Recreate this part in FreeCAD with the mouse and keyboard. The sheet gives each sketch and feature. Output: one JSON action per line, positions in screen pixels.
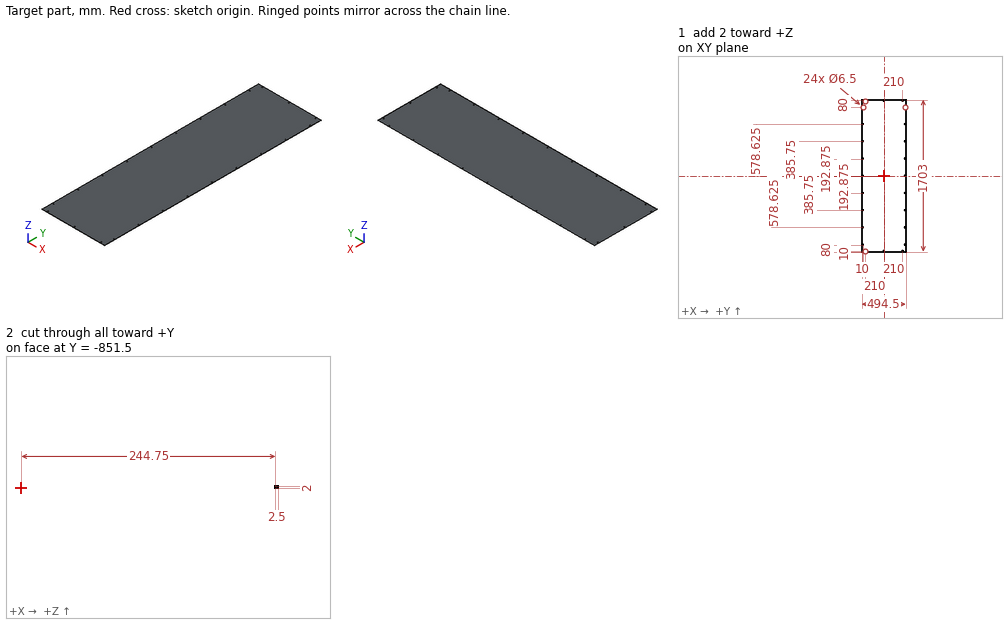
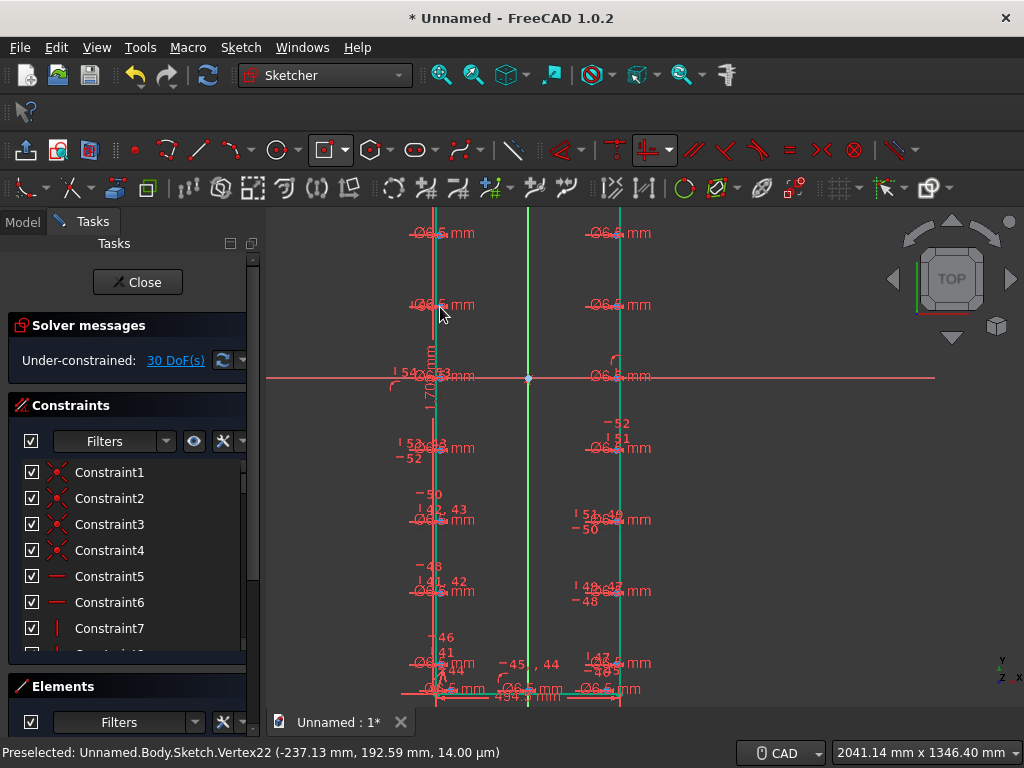
{"action": "left_click", "coordinate": [440, 307]}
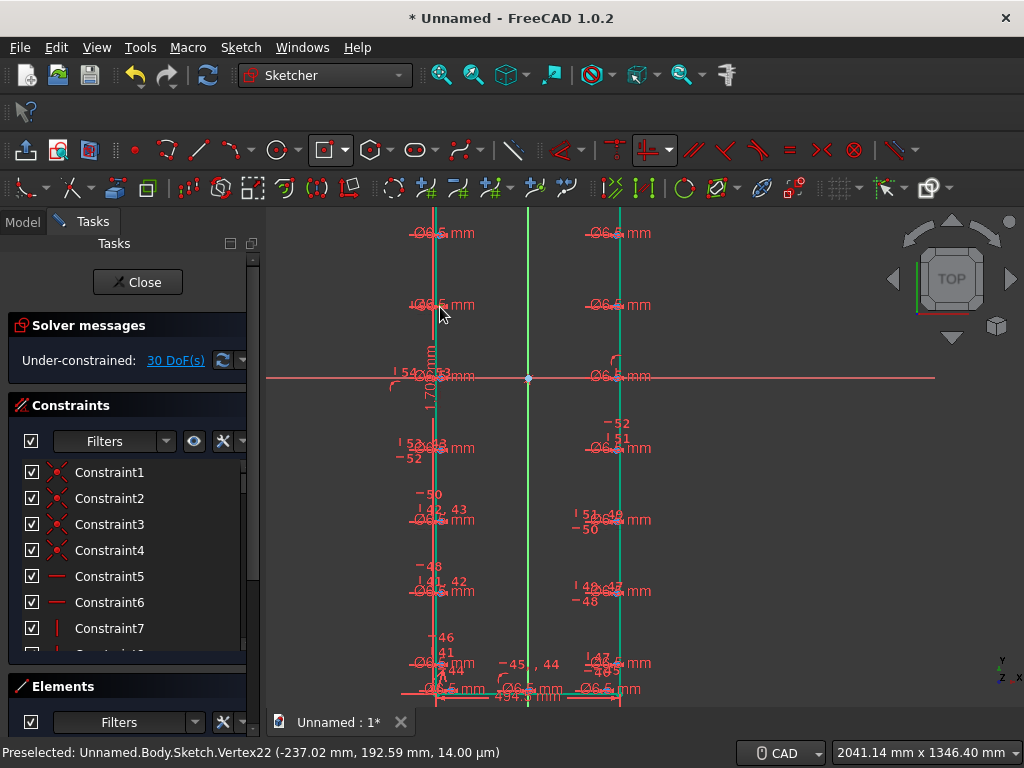
{"action": "left_click", "coordinate": [440, 235]}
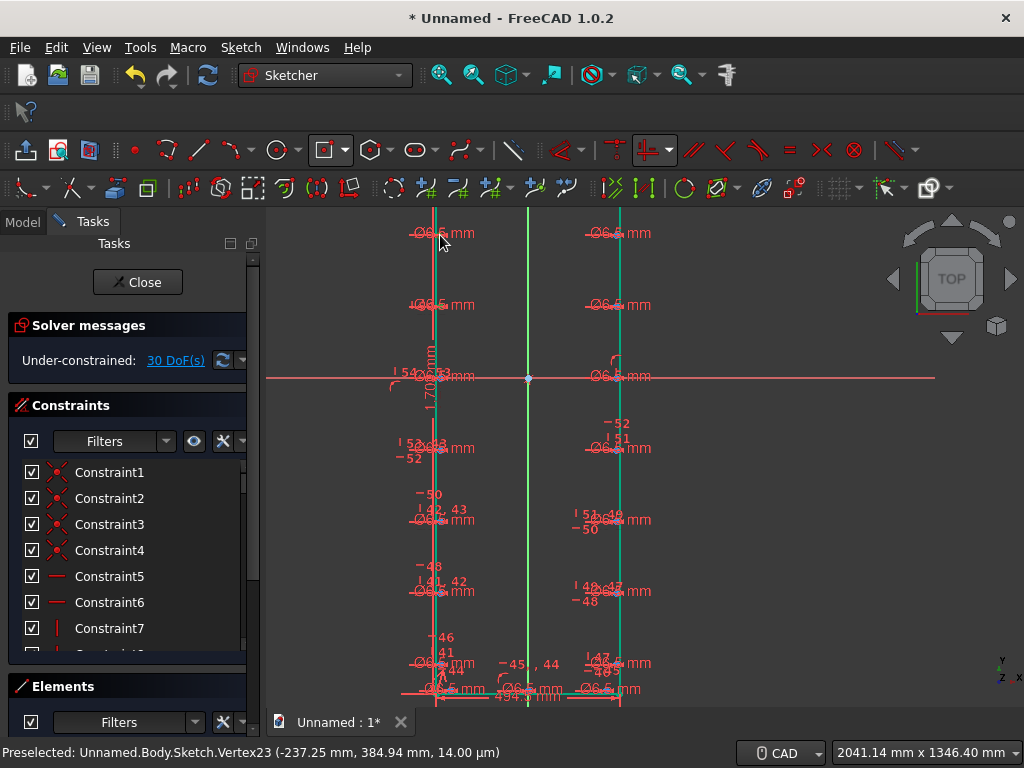
{"action": "key", "text": "v"}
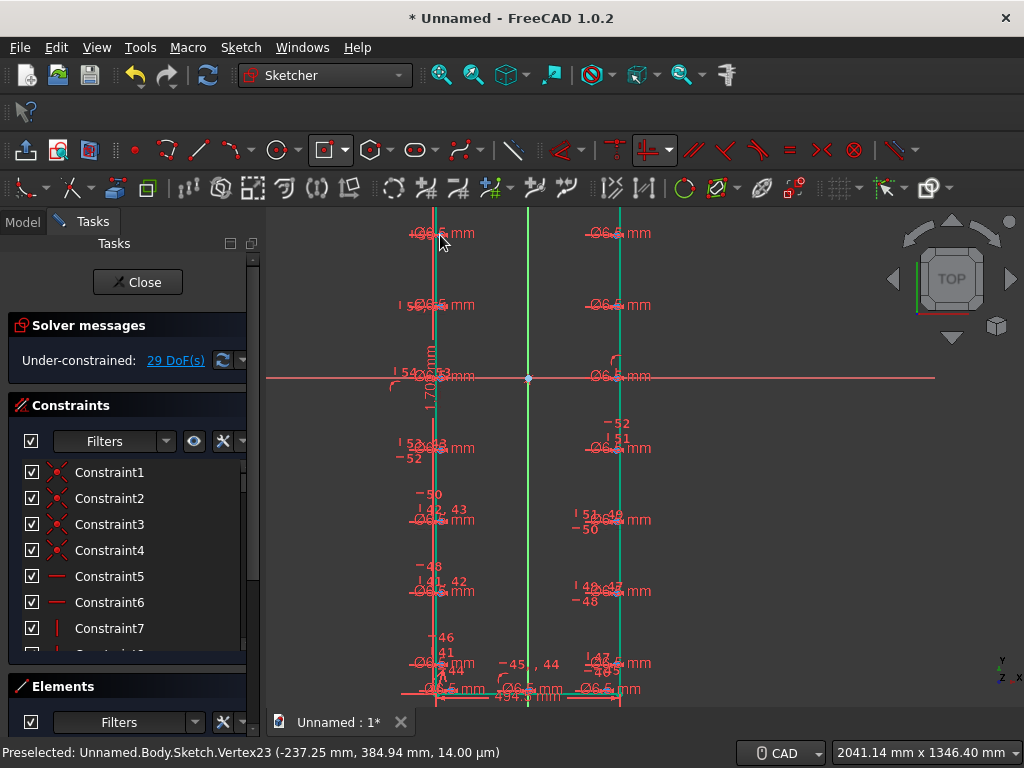
{"action": "left_click", "coordinate": [440, 235]}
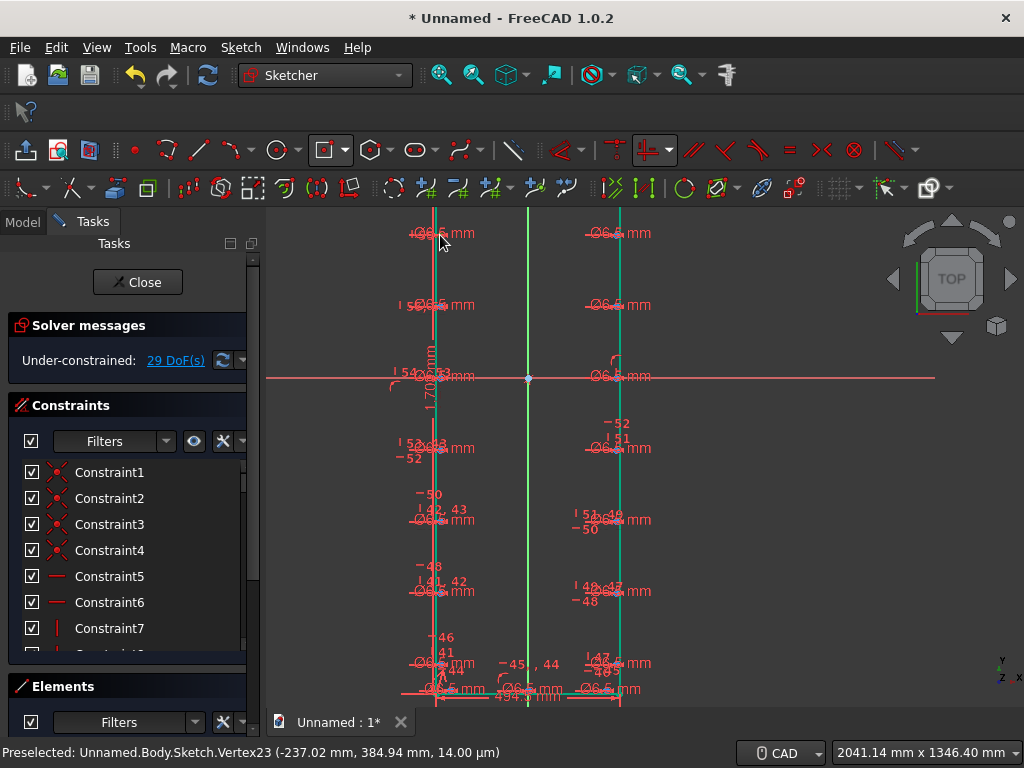
{"action": "scroll", "coordinate": [616, 521], "scroll_direction": "down", "scroll_amount": 4}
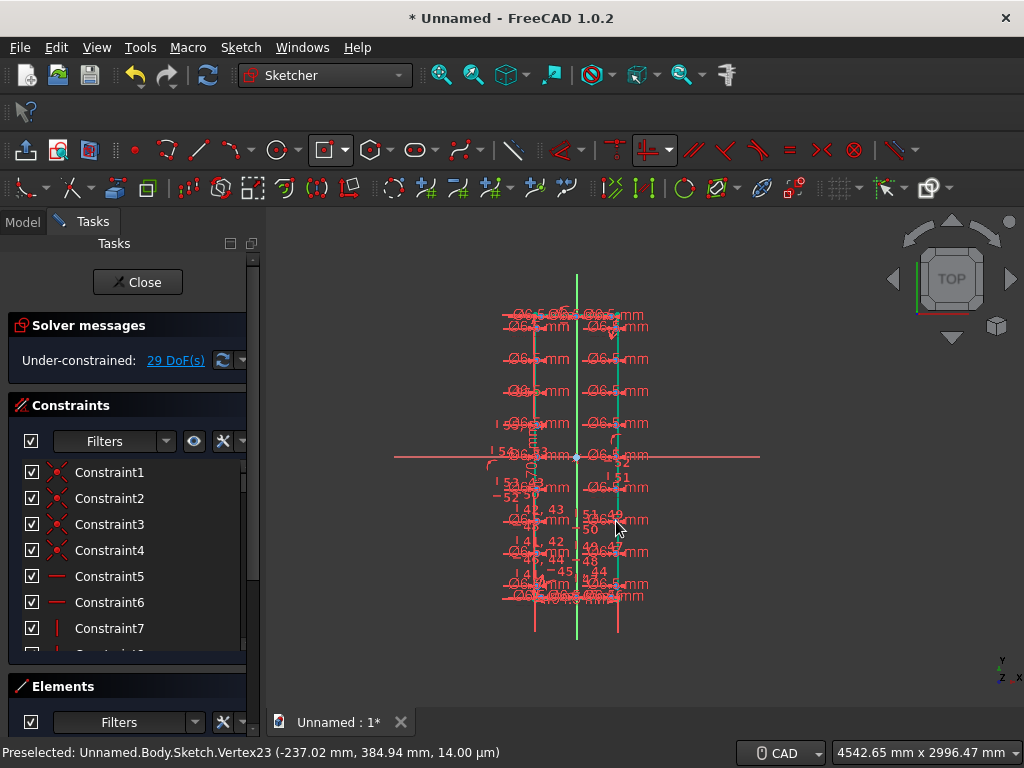
{"action": "left_click", "coordinate": [537, 361]}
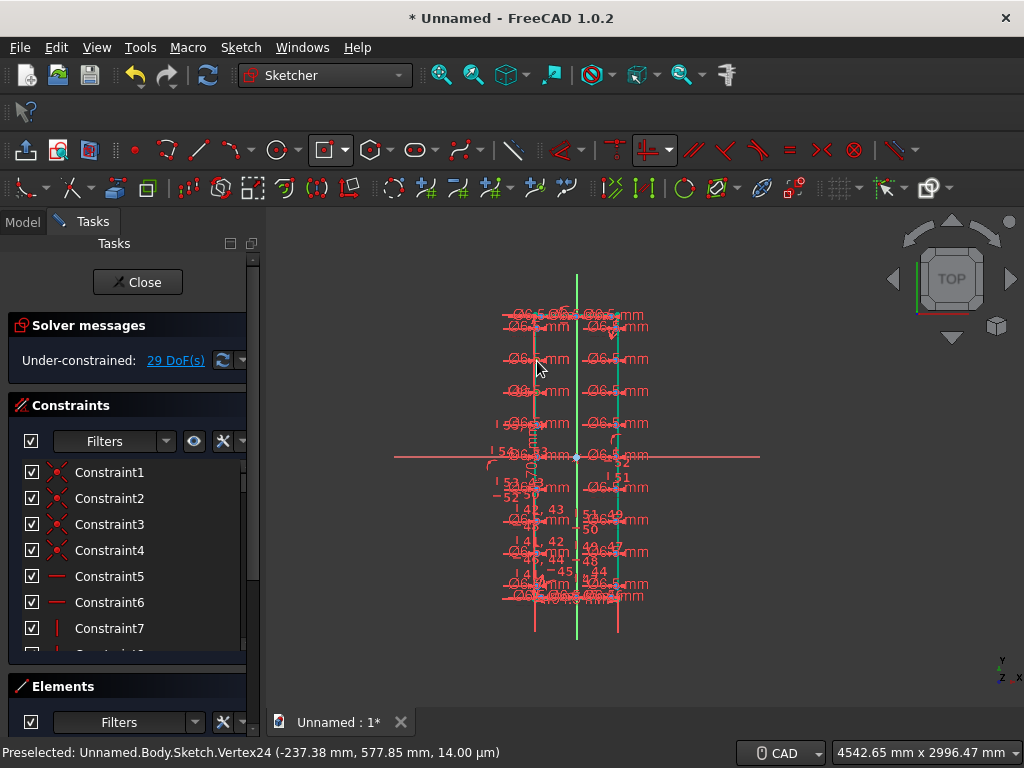
{"action": "key", "text": "v"}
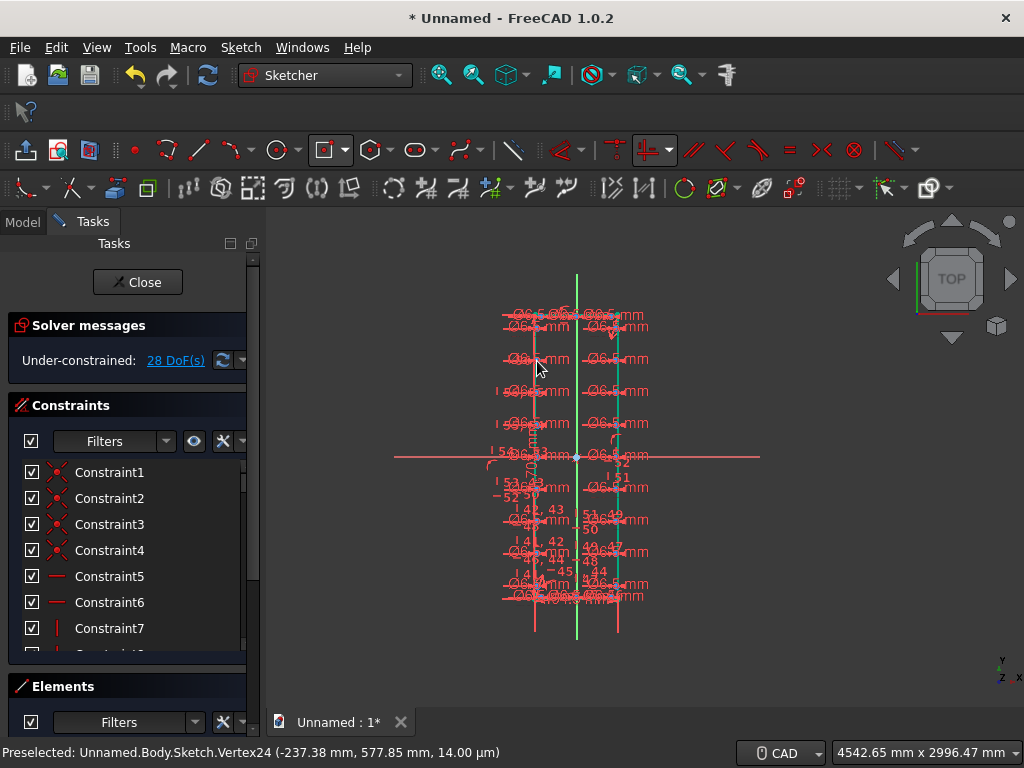
{"action": "left_click", "coordinate": [537, 361]}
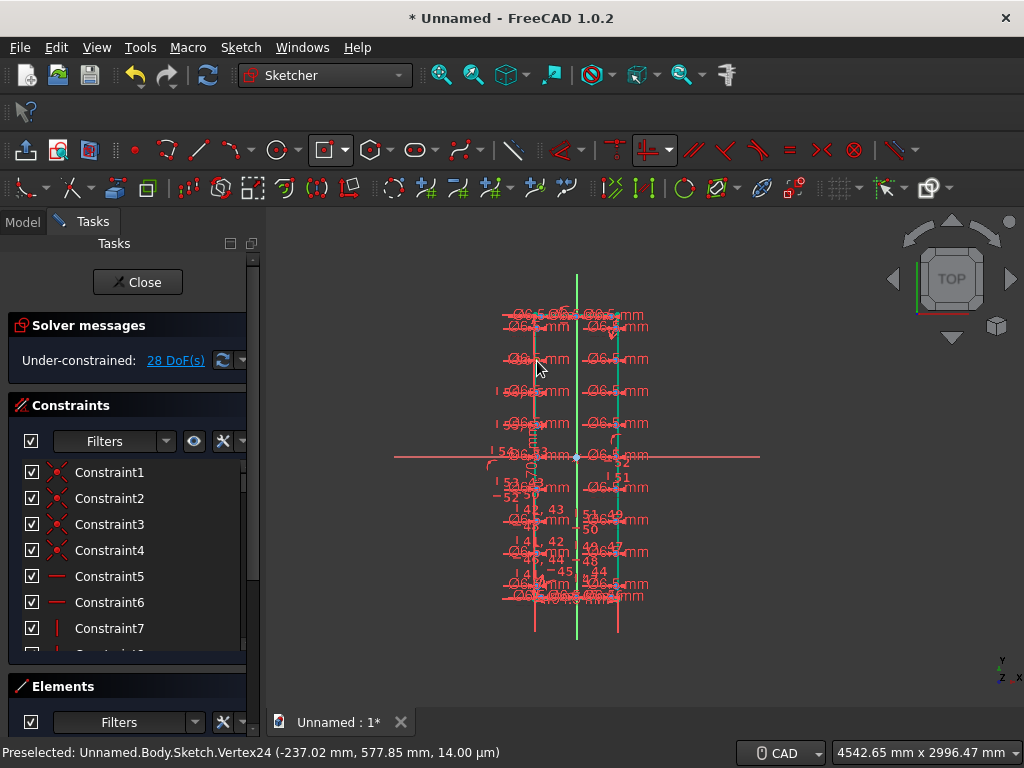
{"action": "left_click", "coordinate": [537, 329]}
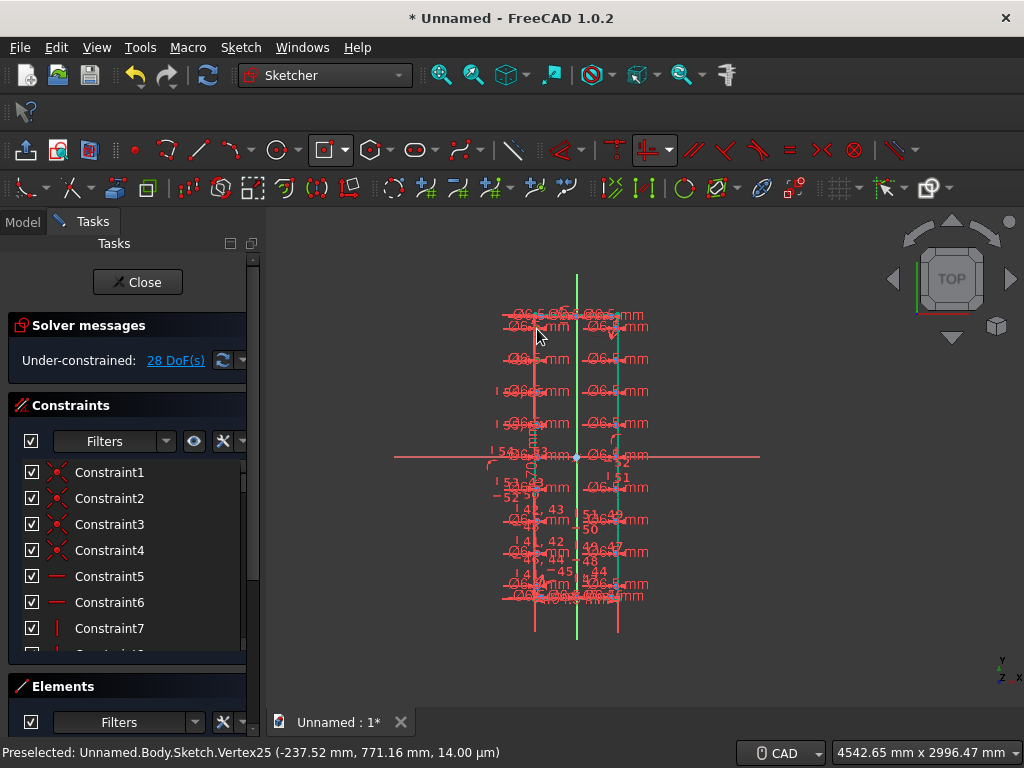
{"action": "left_click", "coordinate": [672, 150]}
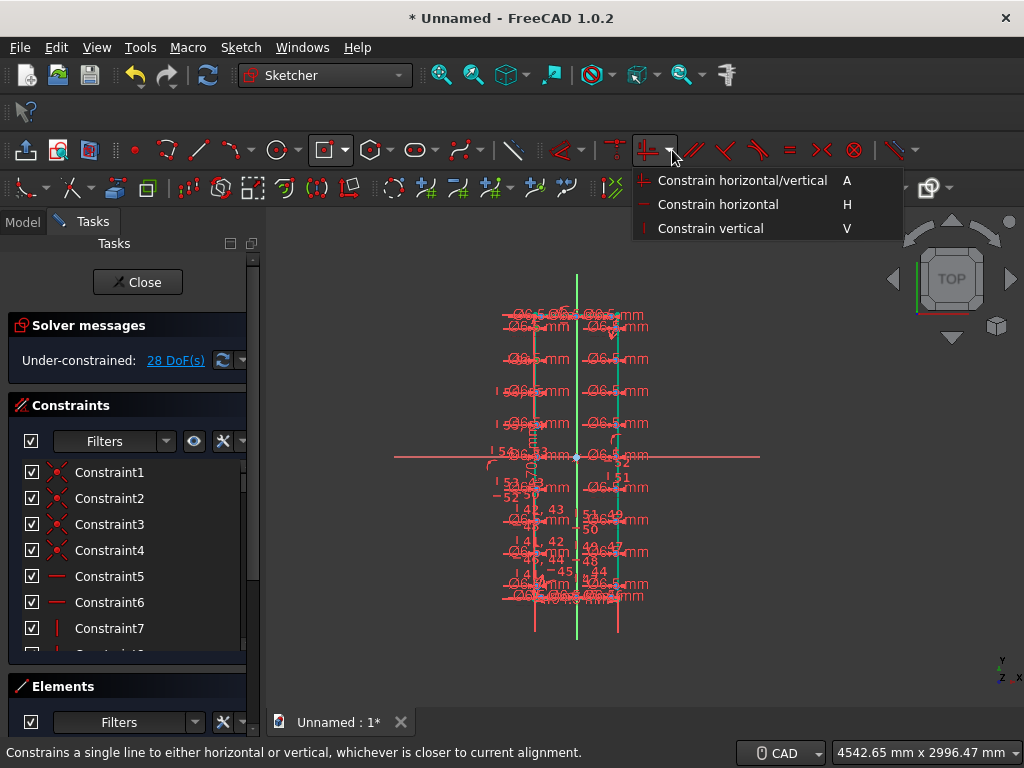
{"action": "left_click", "coordinate": [768, 228]}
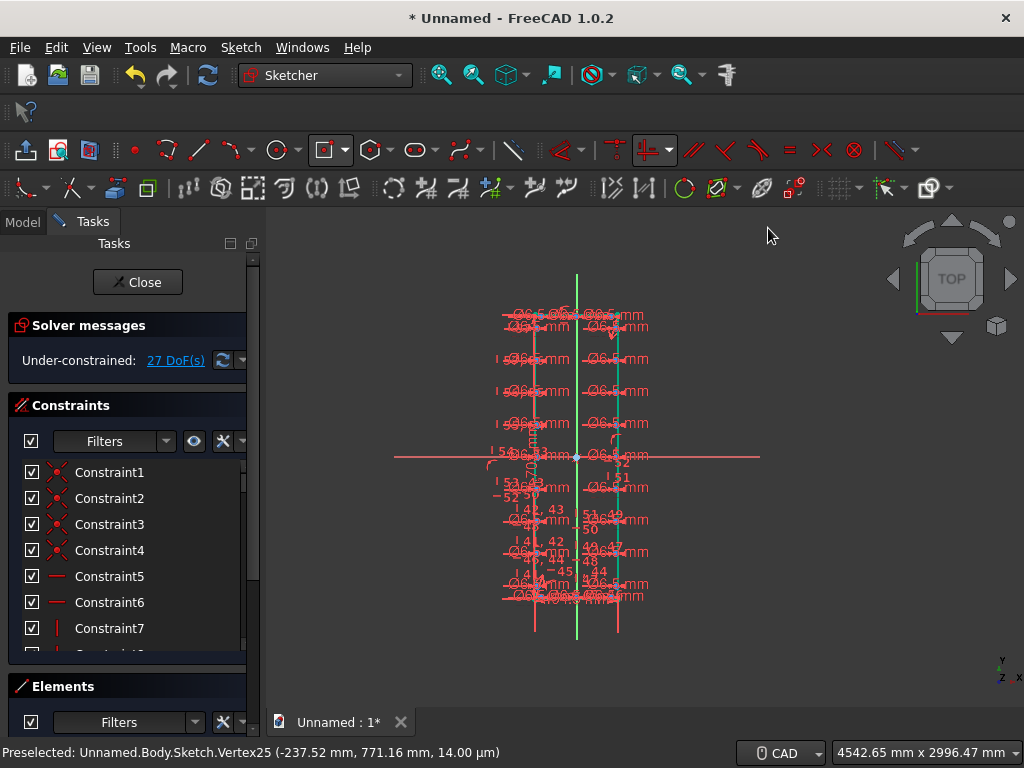
{"action": "left_click", "coordinate": [616, 490]}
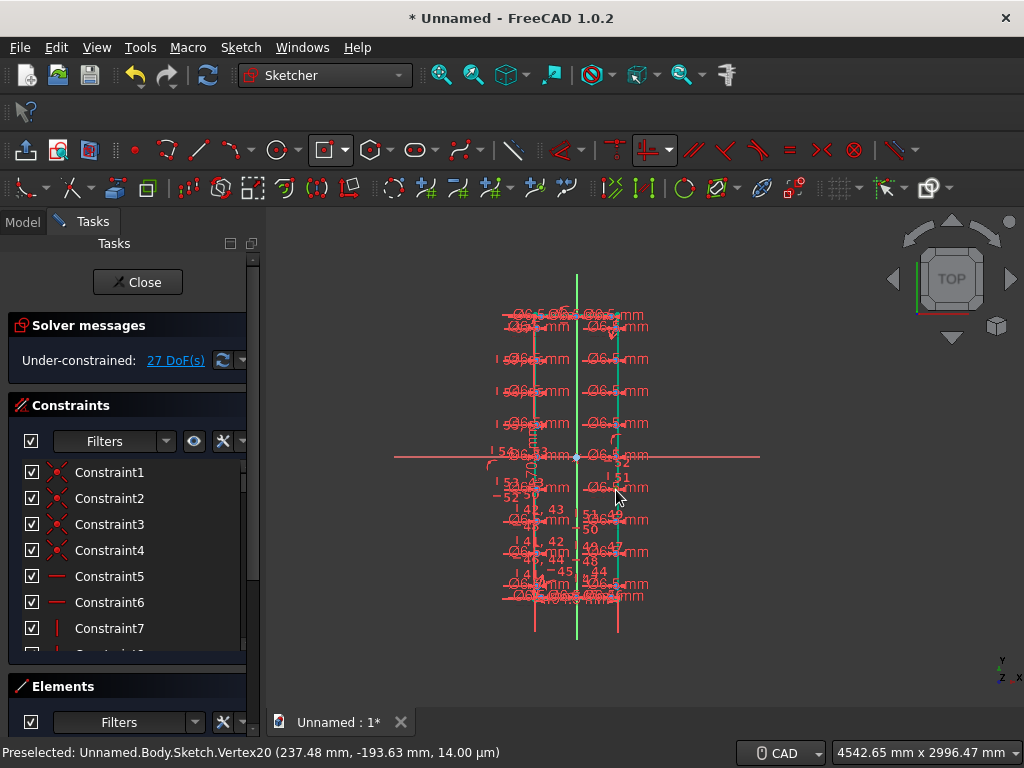
{"action": "scroll", "coordinate": [616, 457], "scroll_direction": "up", "scroll_amount": 4}